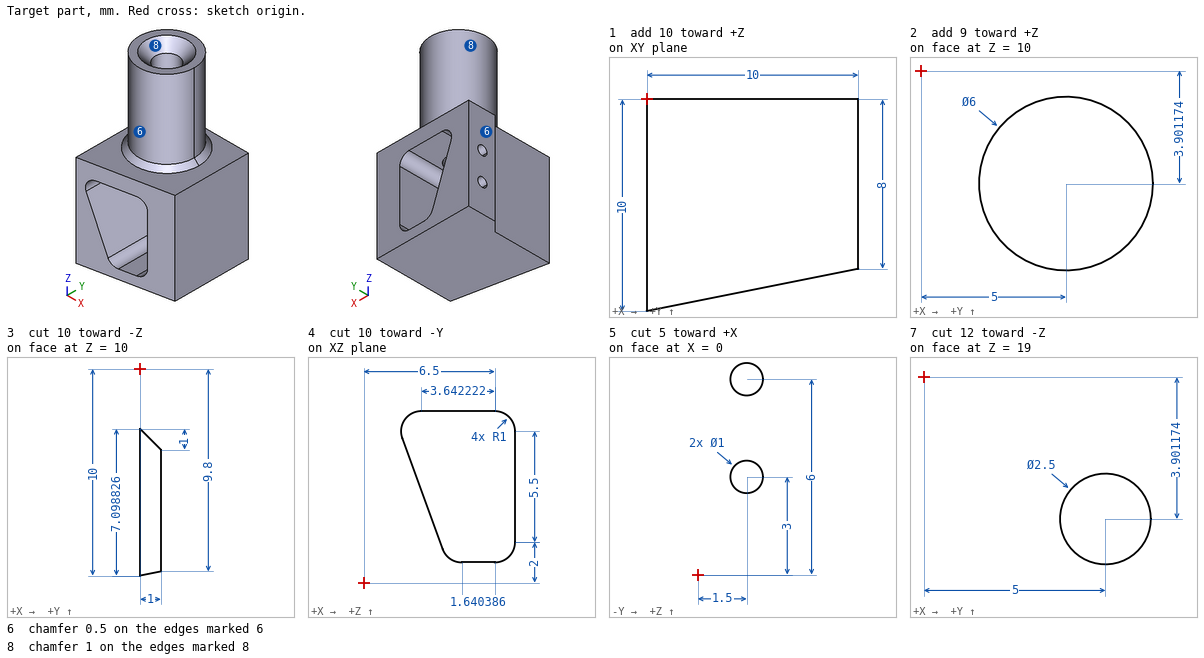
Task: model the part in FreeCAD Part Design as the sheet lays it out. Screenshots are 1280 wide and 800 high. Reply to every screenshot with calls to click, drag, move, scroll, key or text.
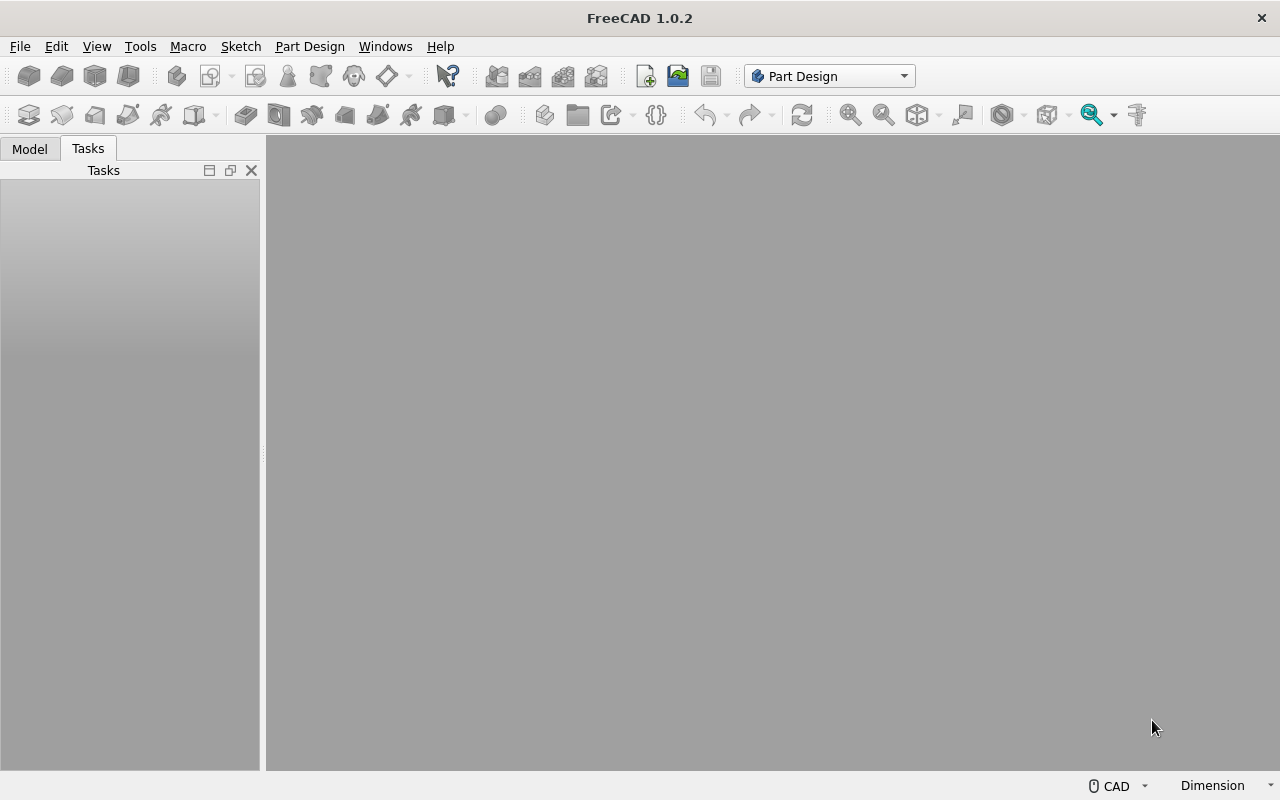
key(ctrl+n)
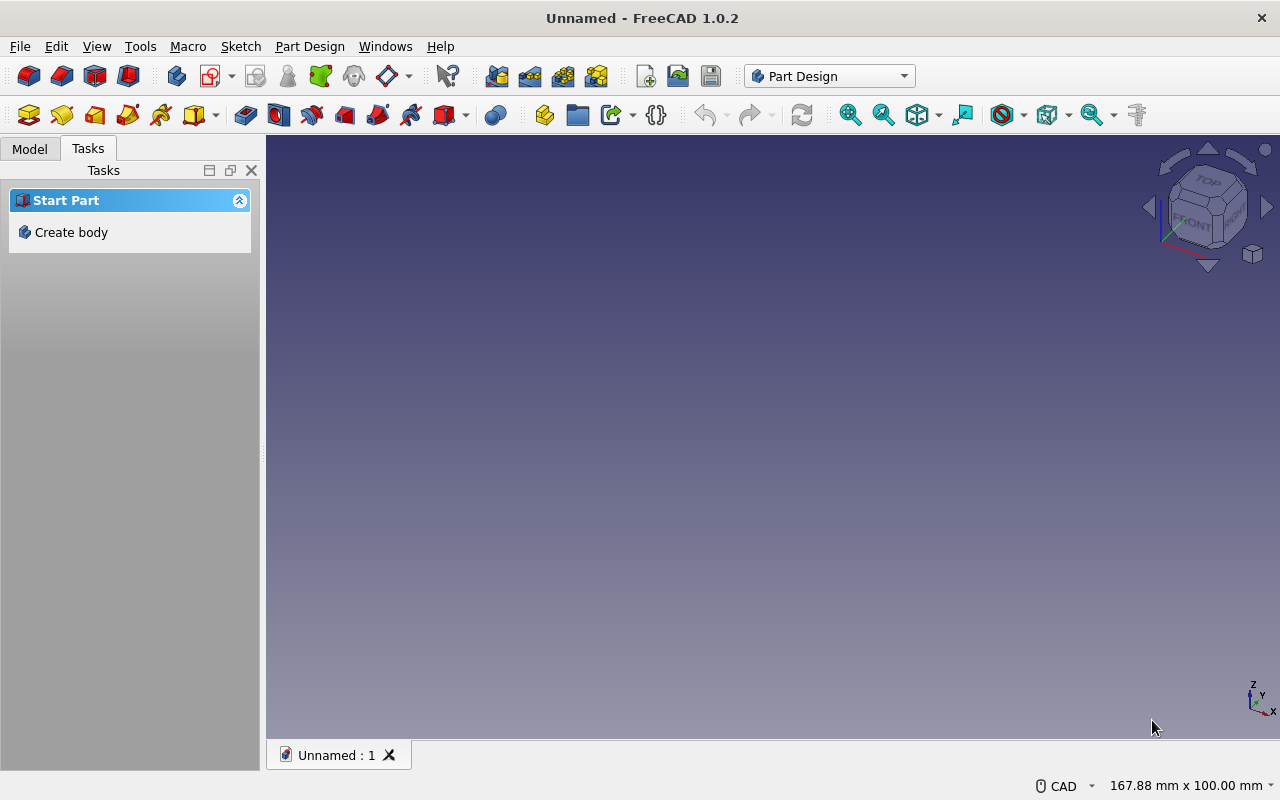
click(210, 76)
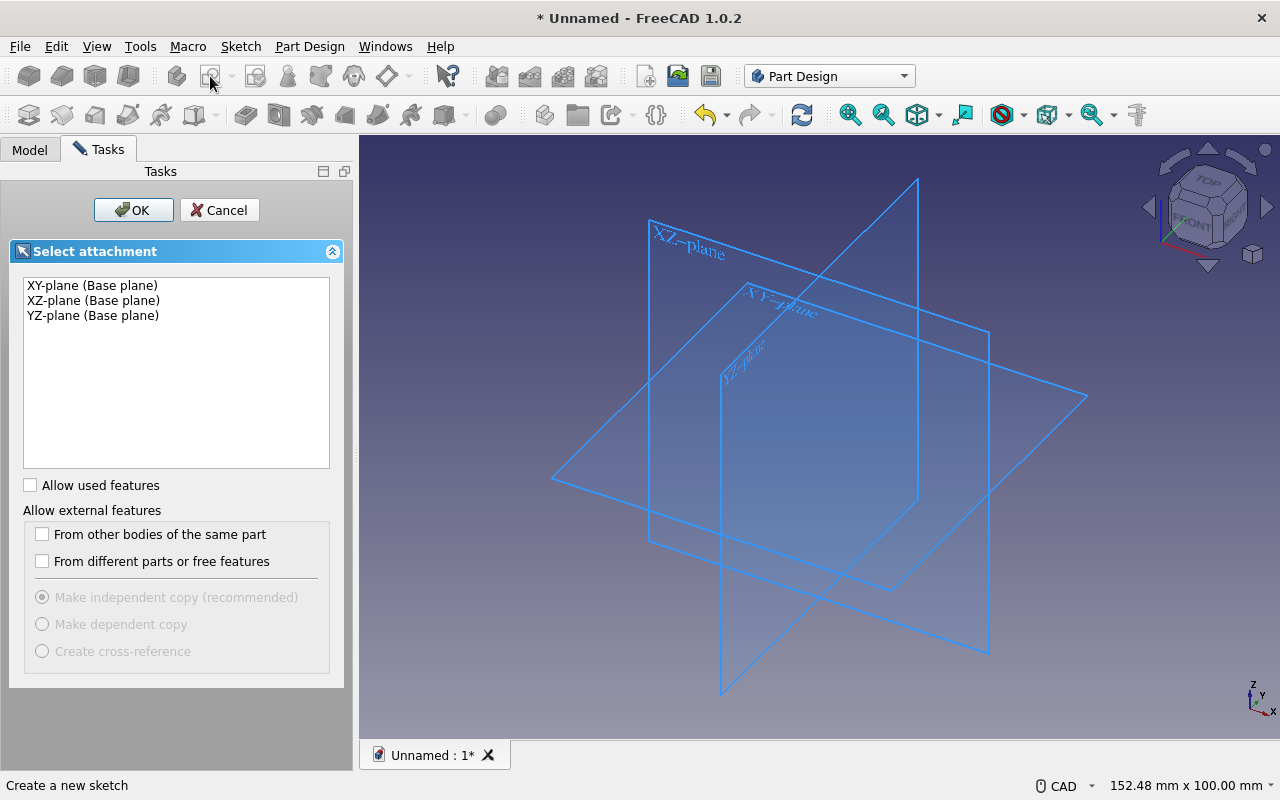
click(84, 286)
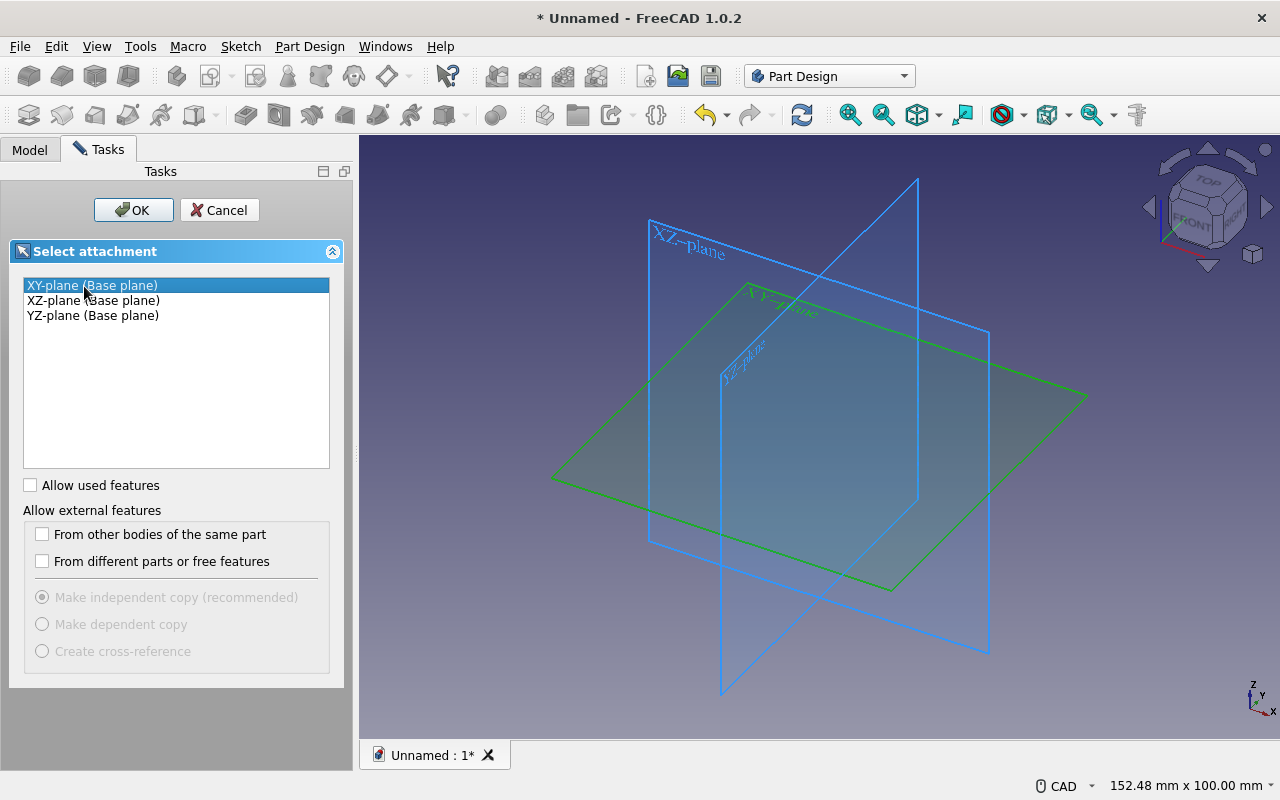
click(134, 210)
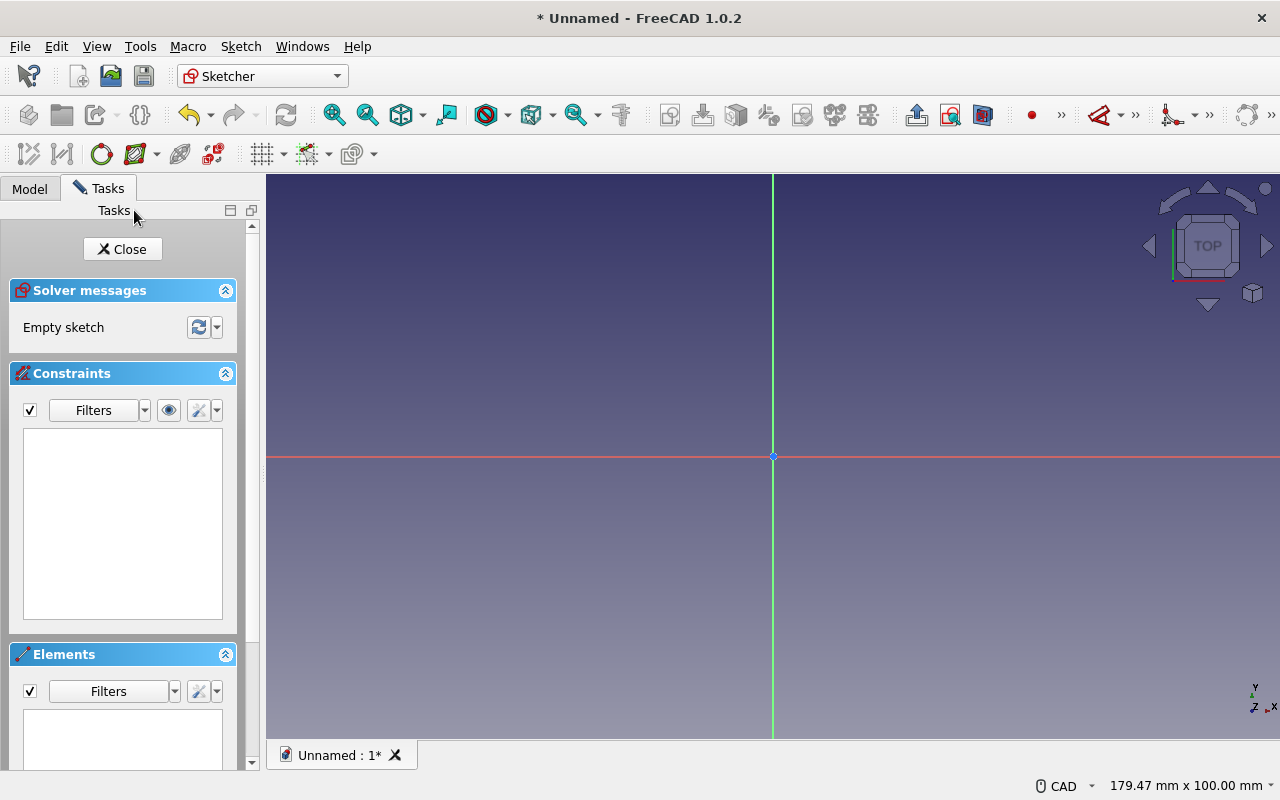
scroll(820, 490, up, 9)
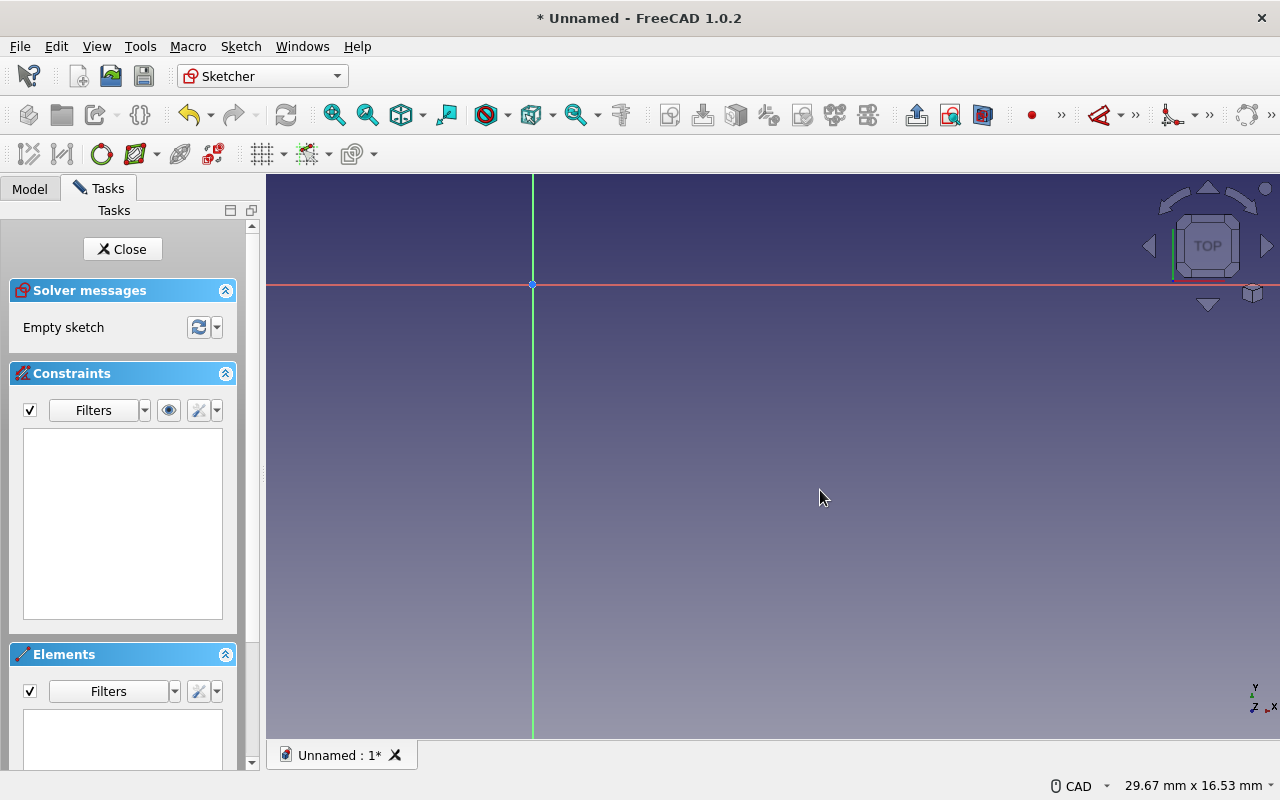
key(g)
key(m)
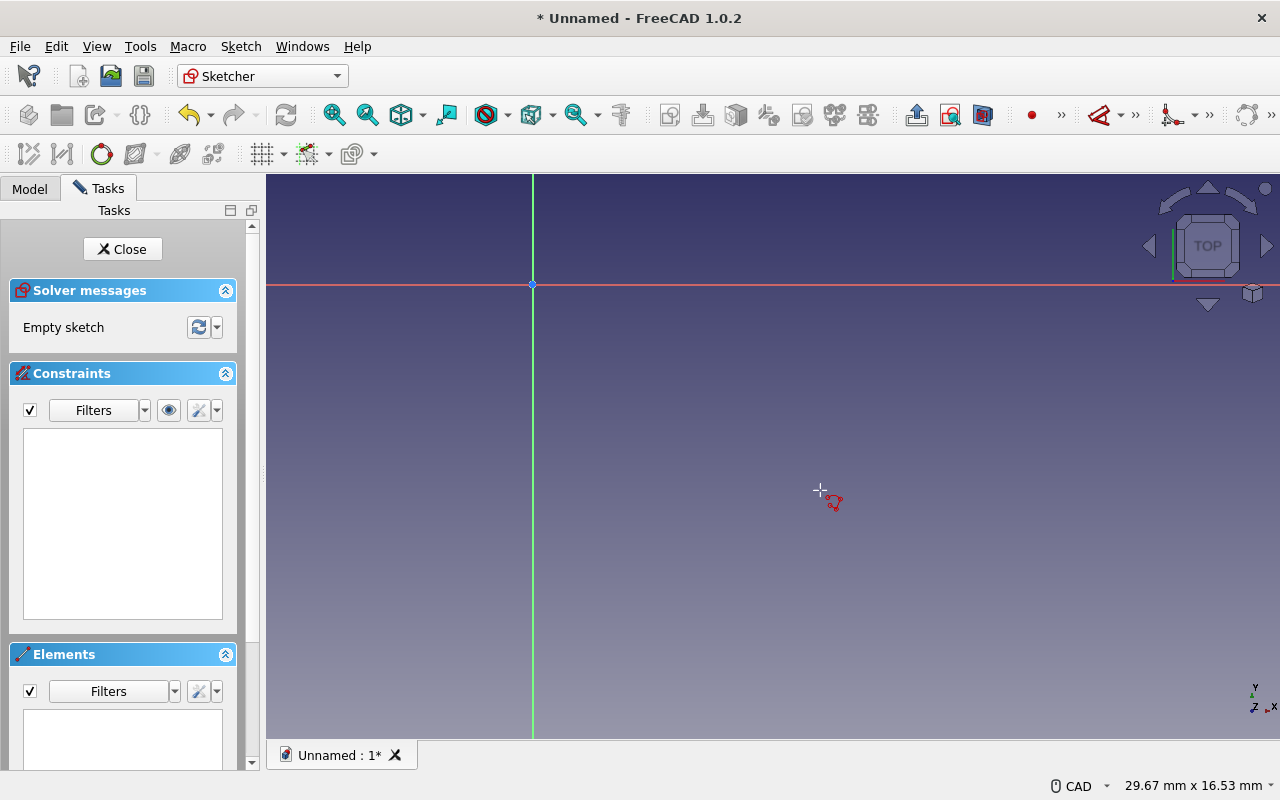
click(533, 285)
click(542, 626)
click(875, 558)
click(875, 294)
click(533, 285)
key(Escape)
key(Escape)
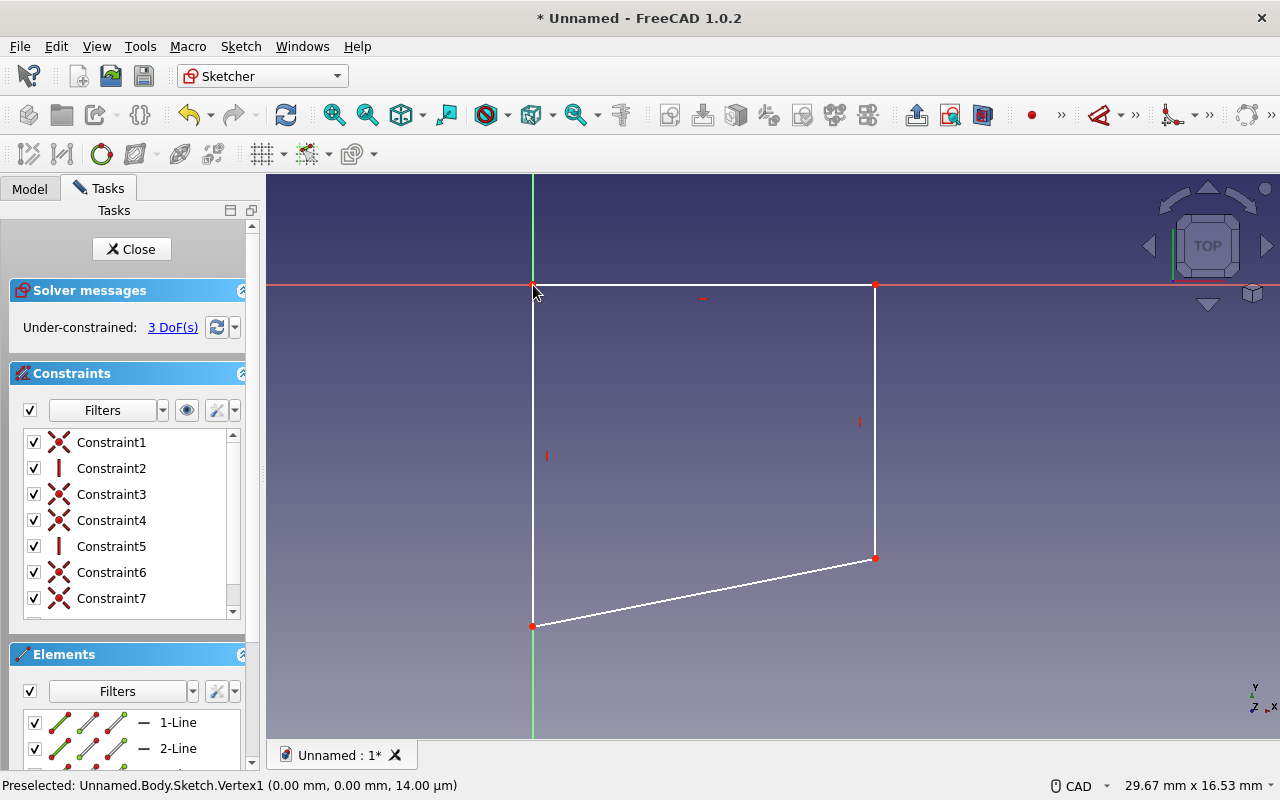
key(d)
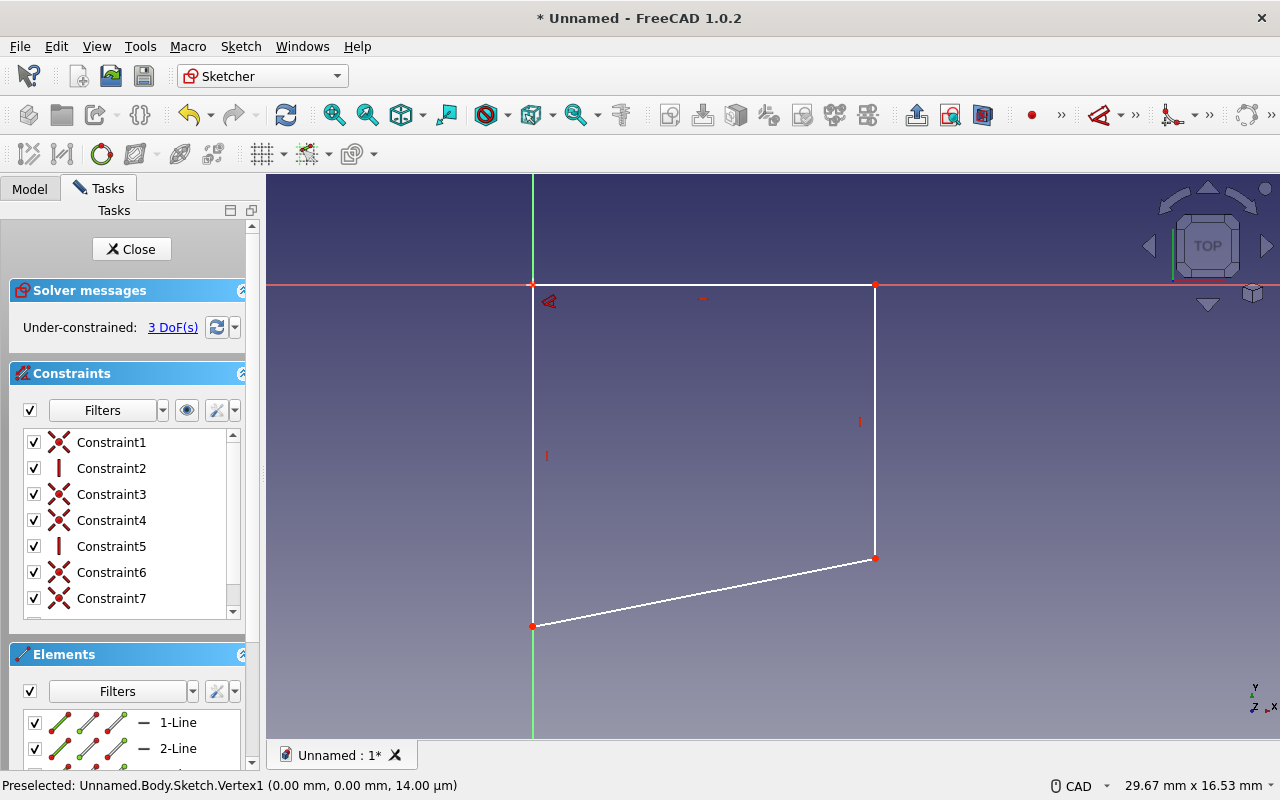
click(875, 477)
click(909, 422)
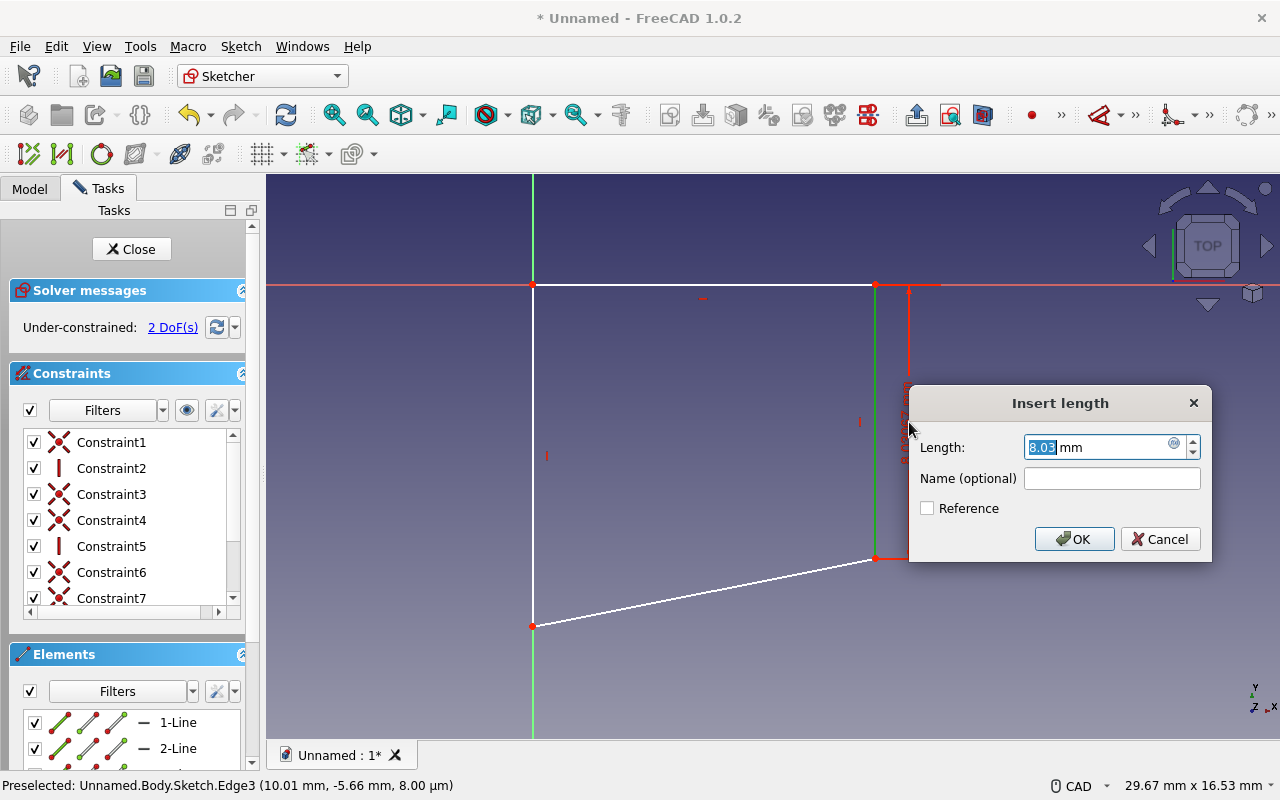
text(8)
key(Return)